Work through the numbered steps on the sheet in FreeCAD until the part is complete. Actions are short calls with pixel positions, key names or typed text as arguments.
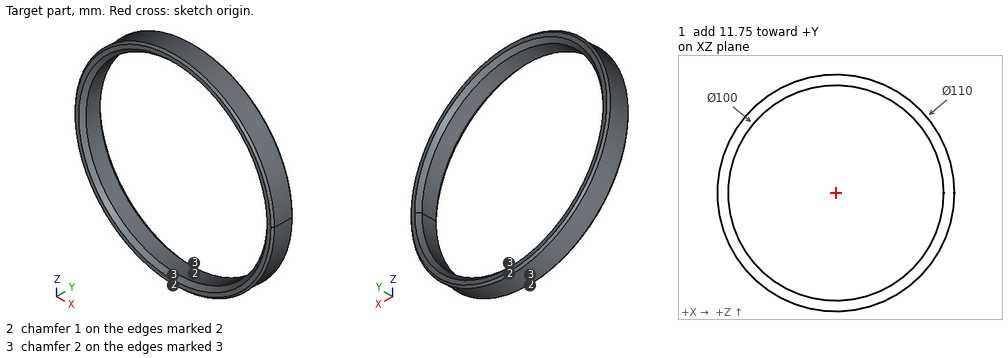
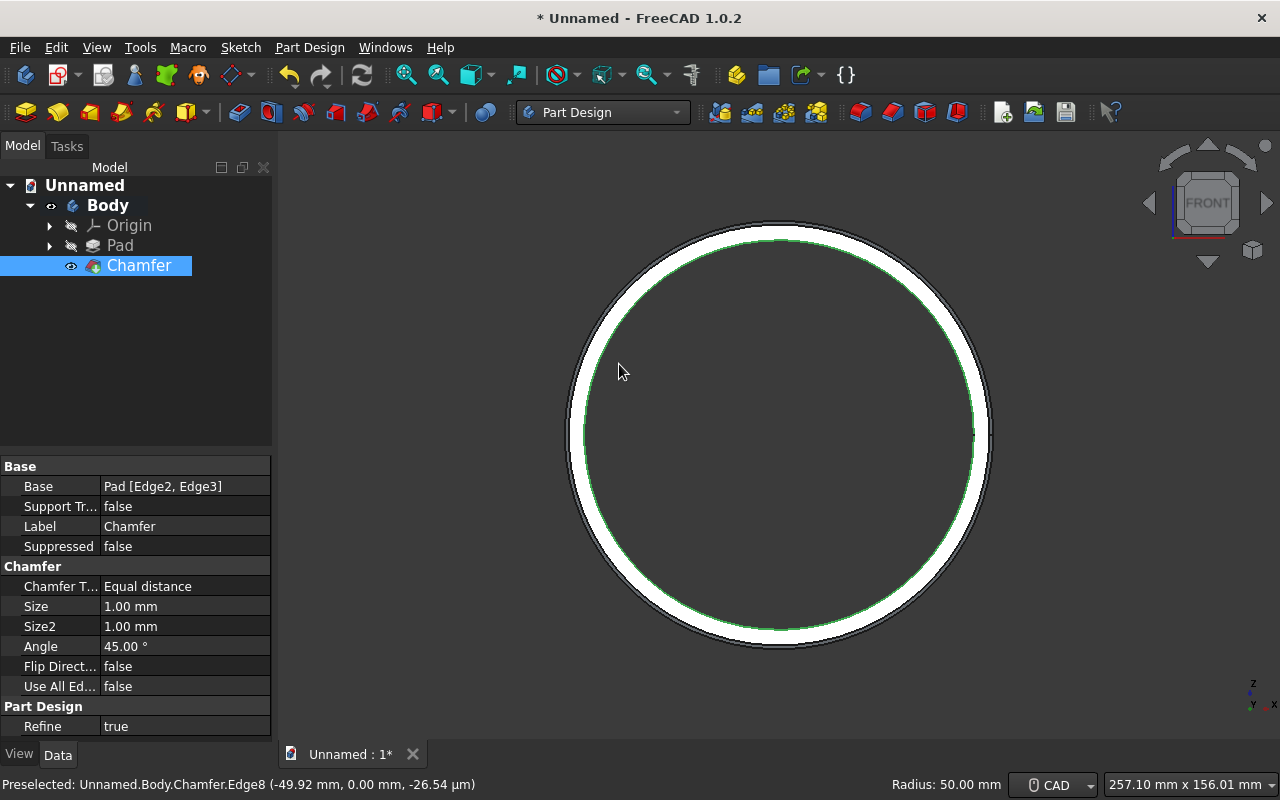
key(3)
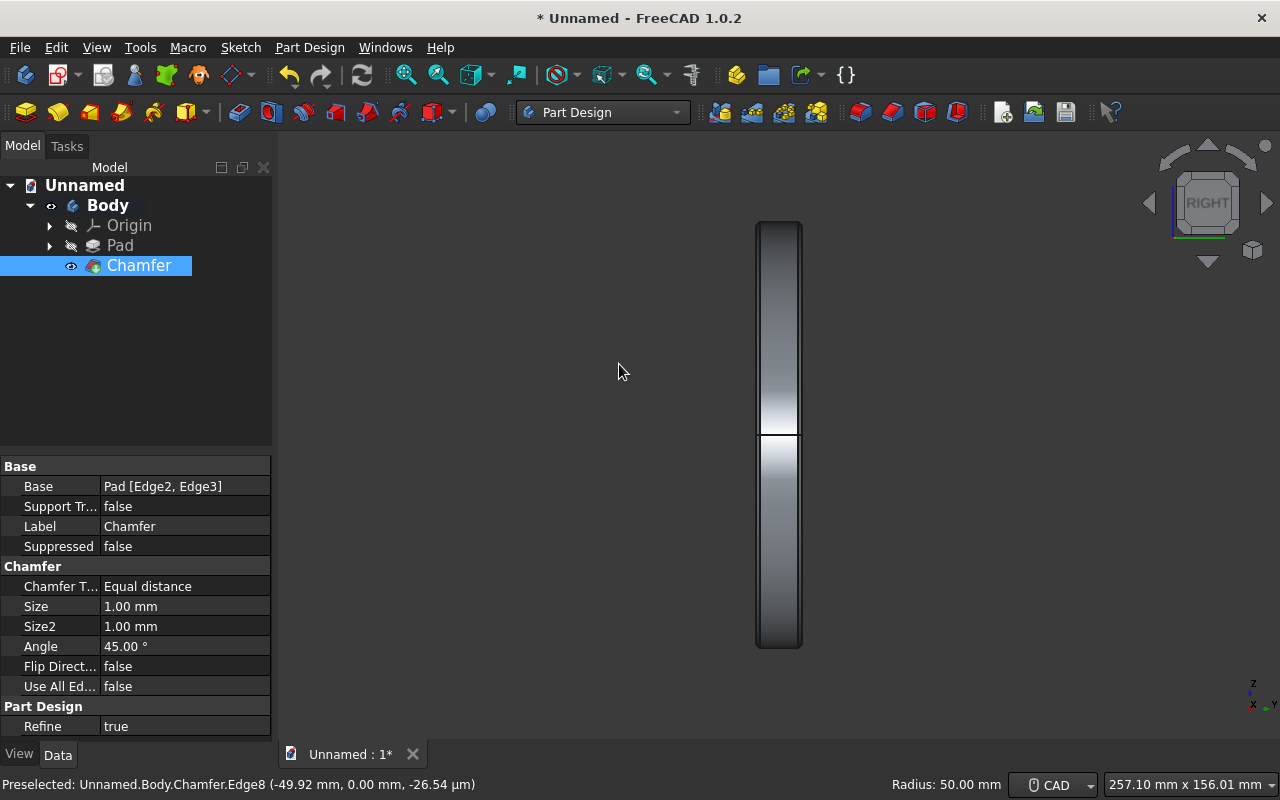
key(5)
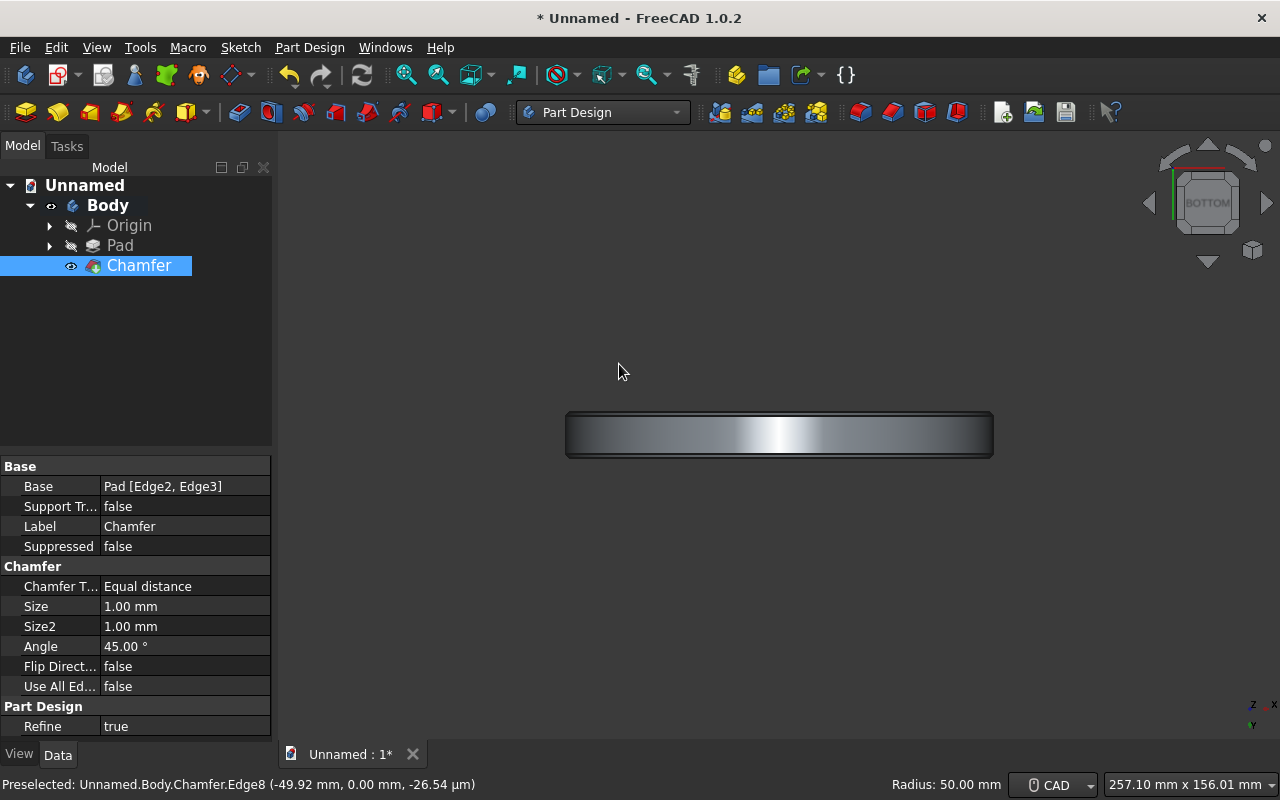
click(408, 76)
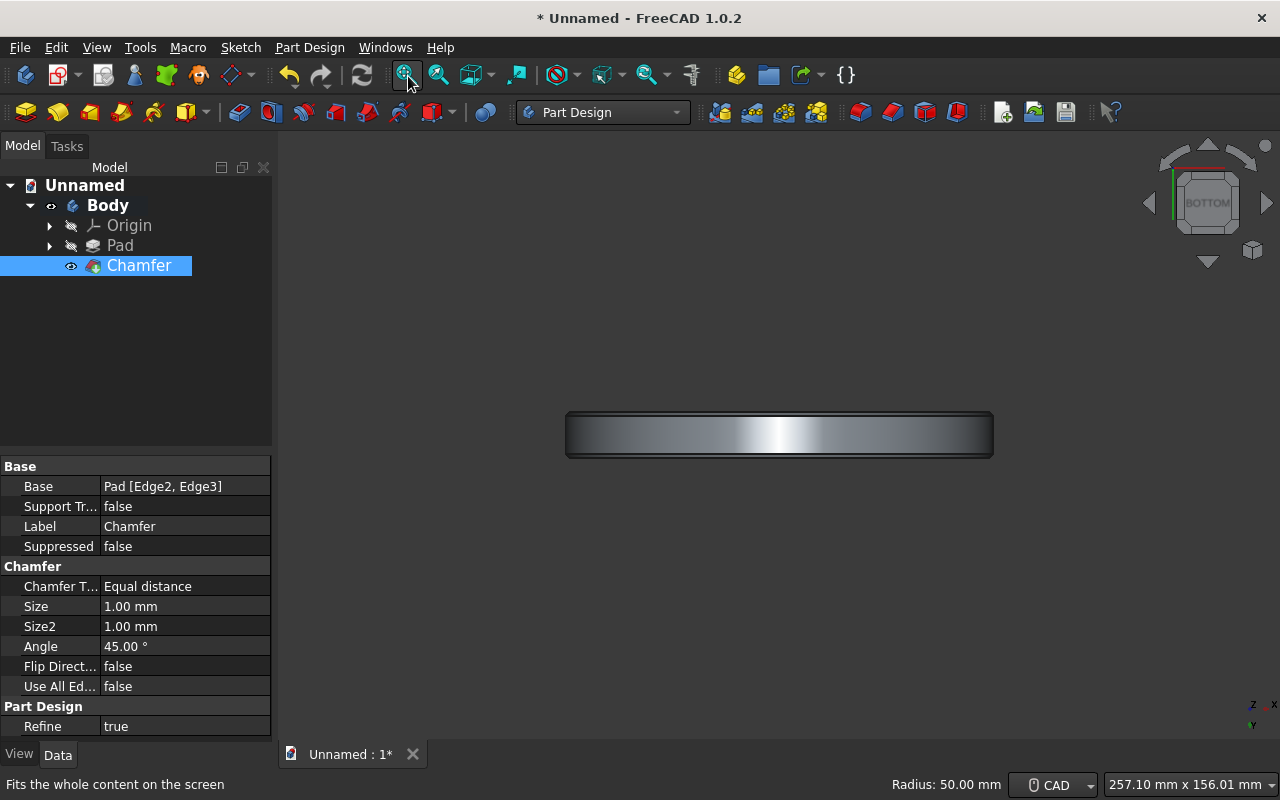
key(4)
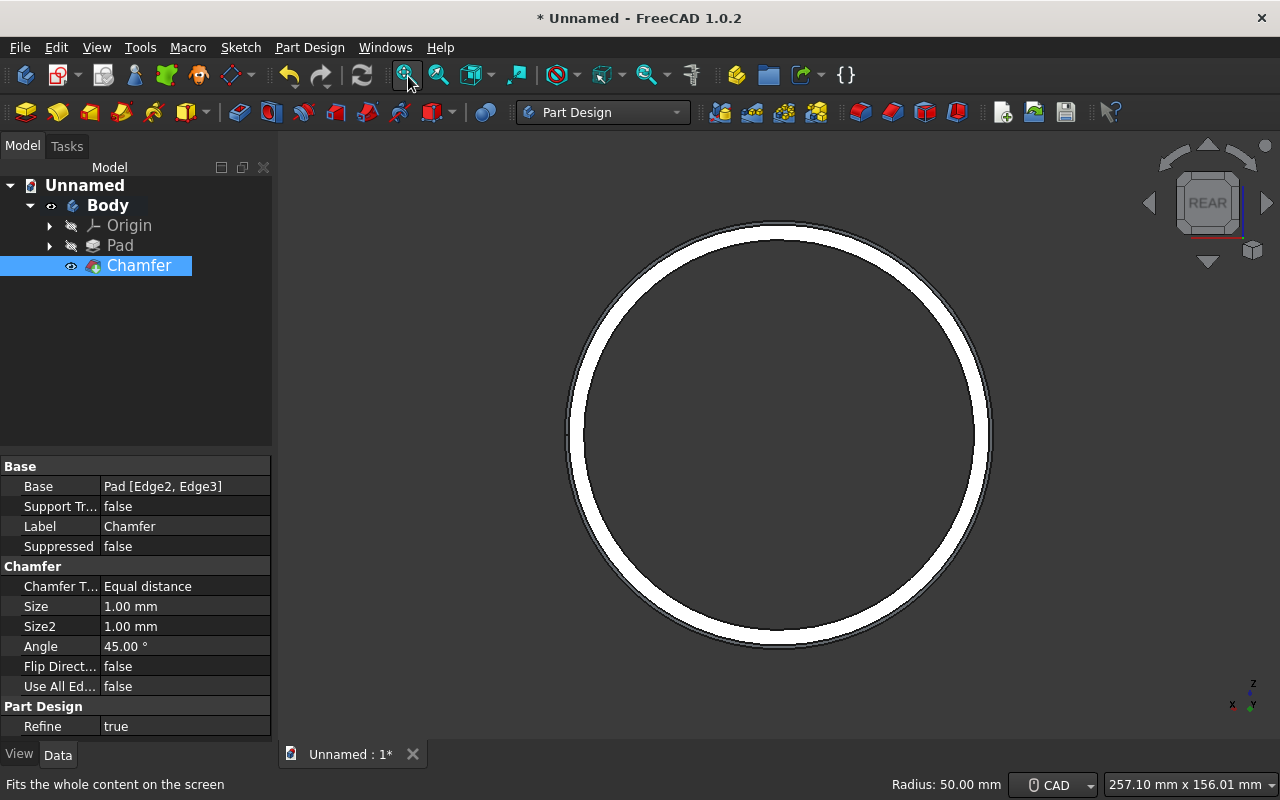
click(974, 434, ctrl)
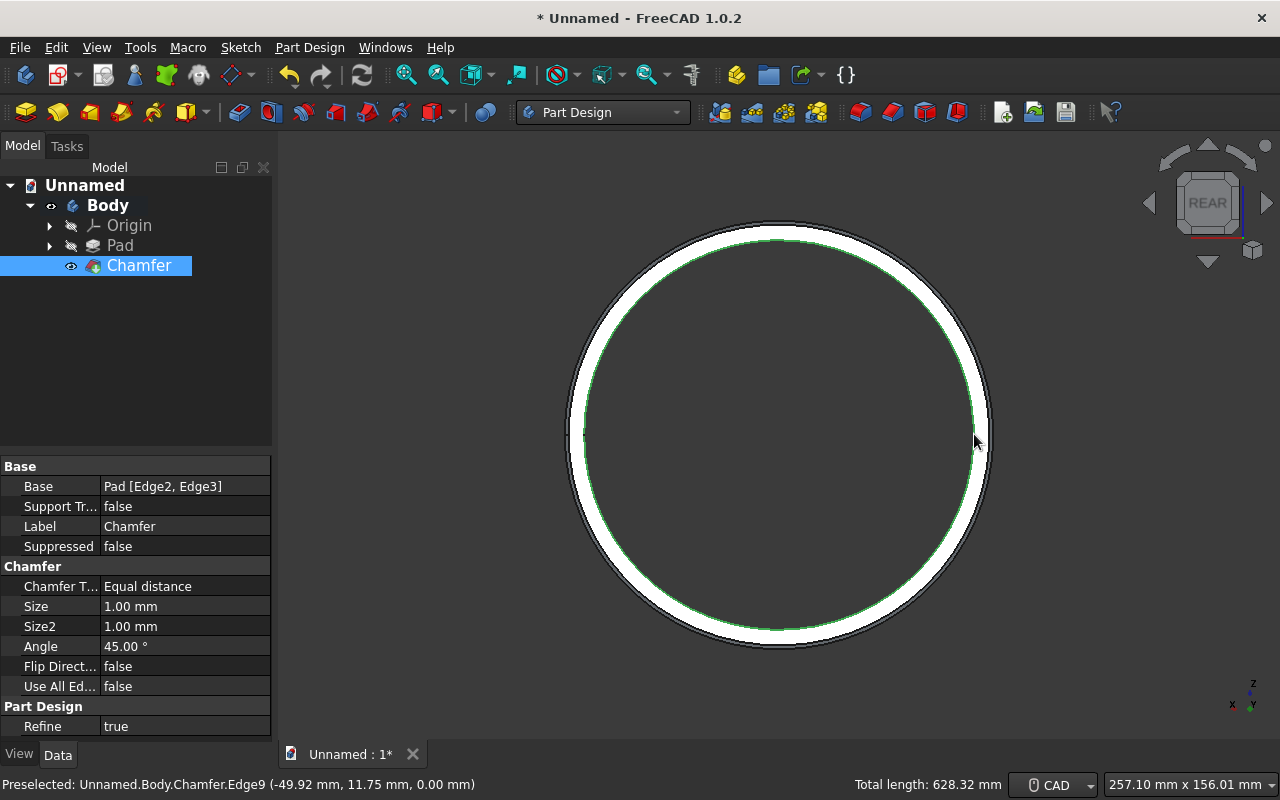
click(894, 112)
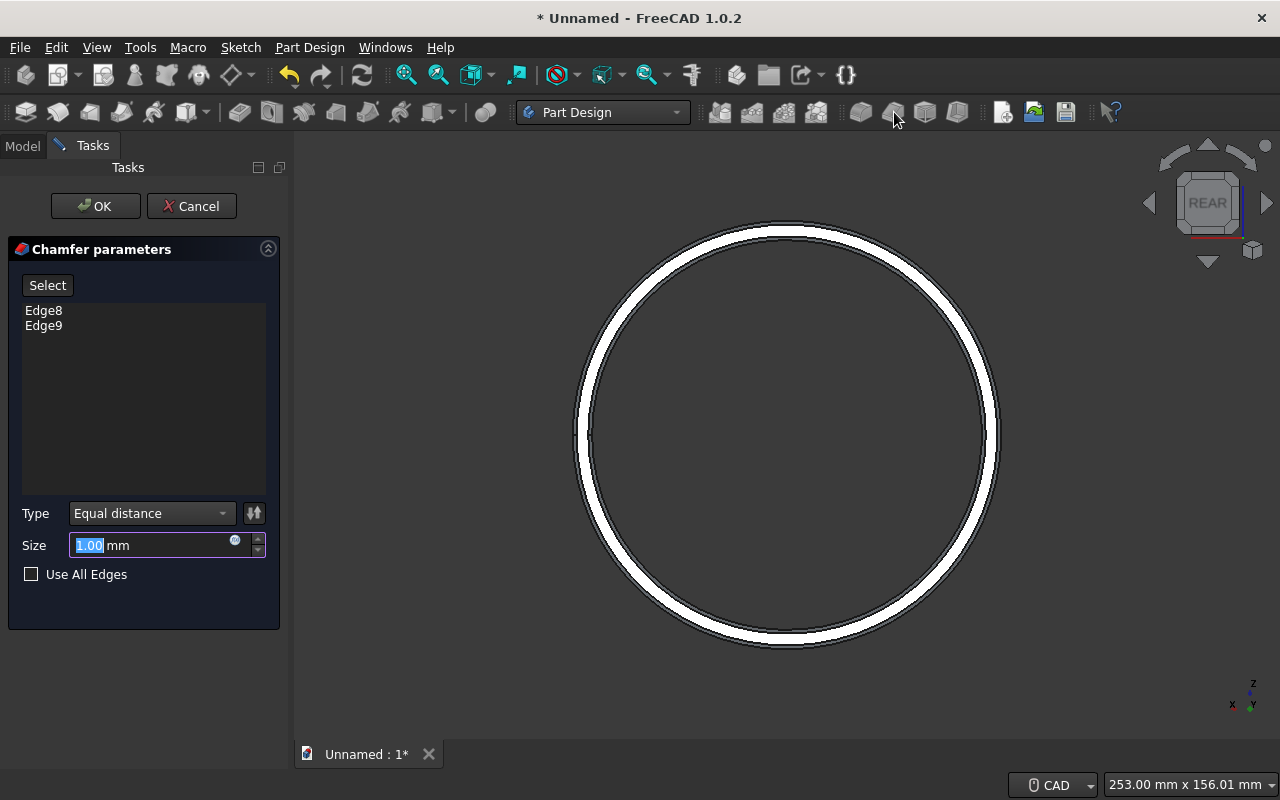
text(2)
key(Tab)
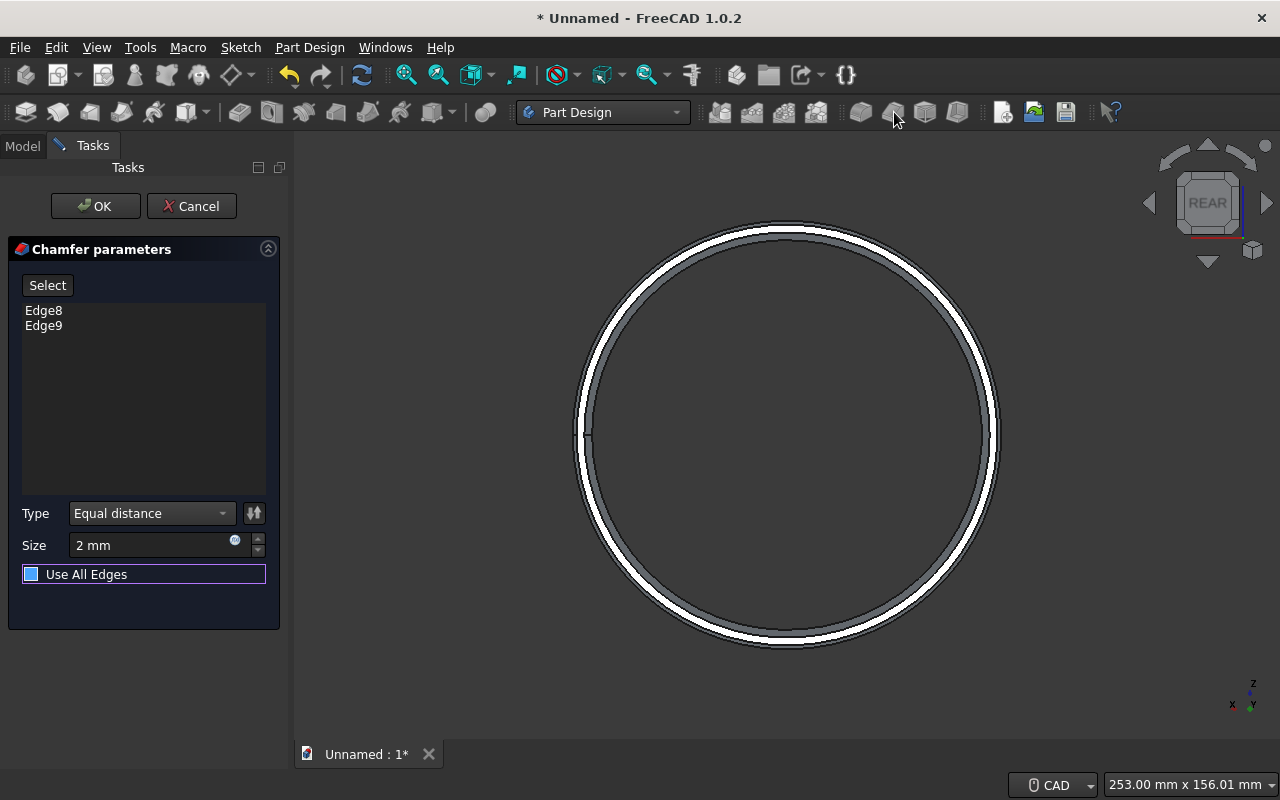
click(96, 206)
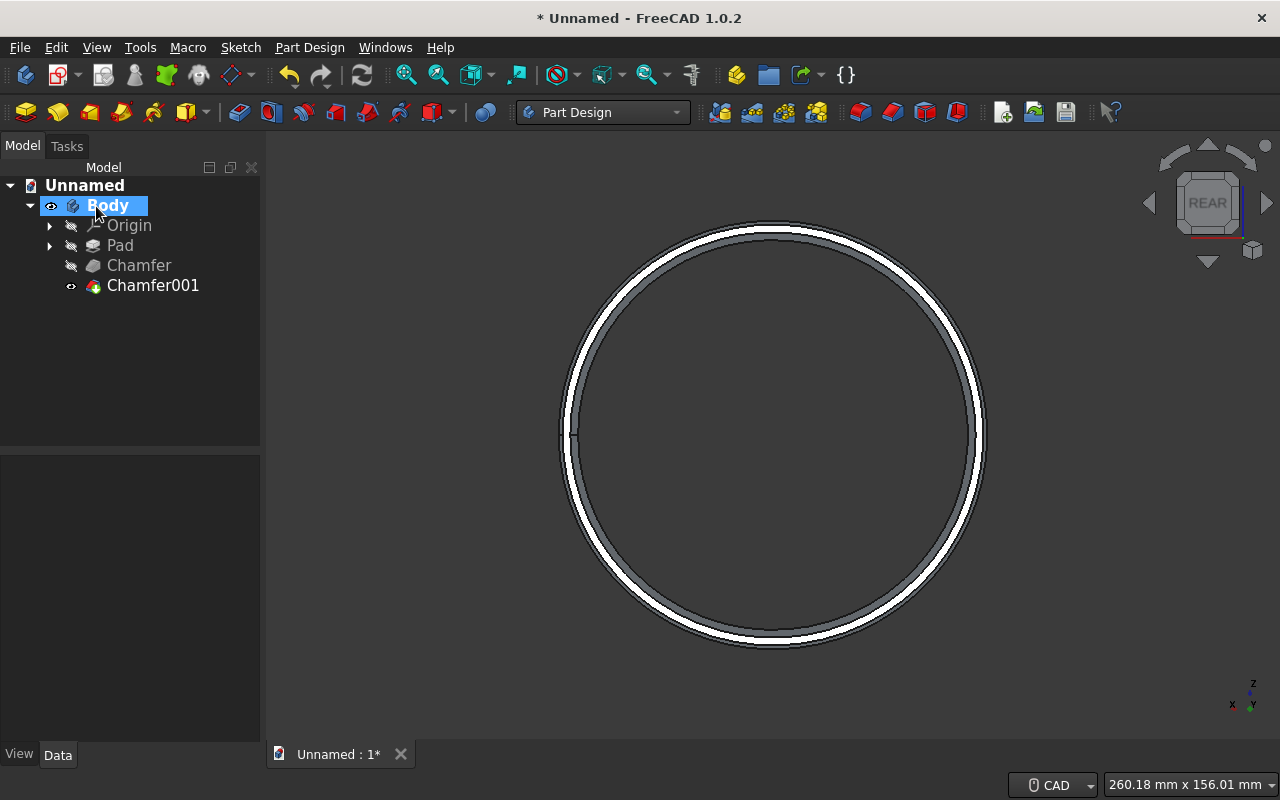
key(0)